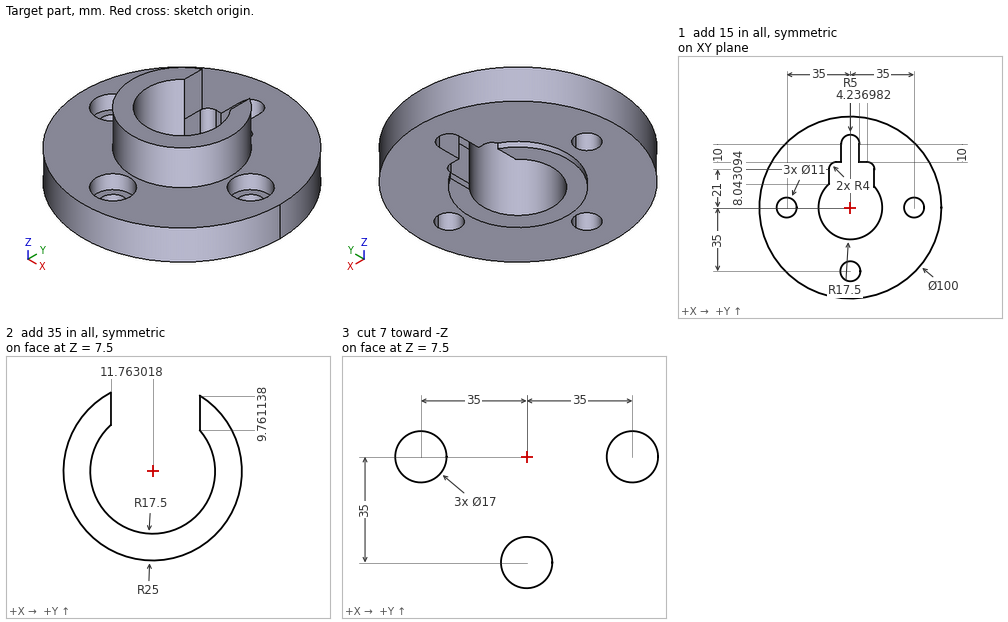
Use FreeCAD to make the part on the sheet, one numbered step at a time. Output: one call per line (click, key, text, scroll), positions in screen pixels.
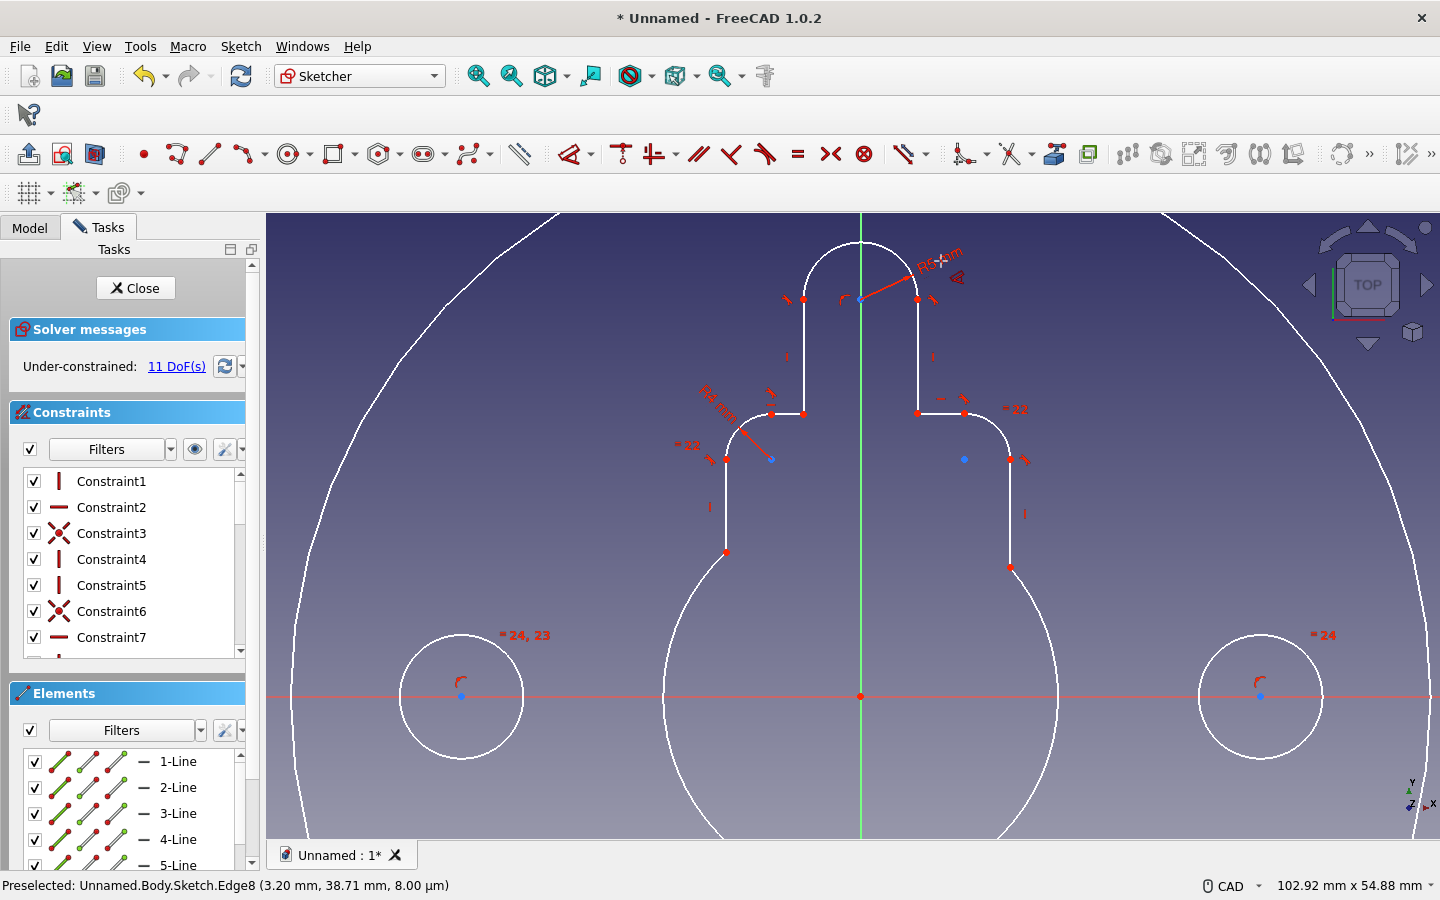
click(696, 805)
click(632, 715)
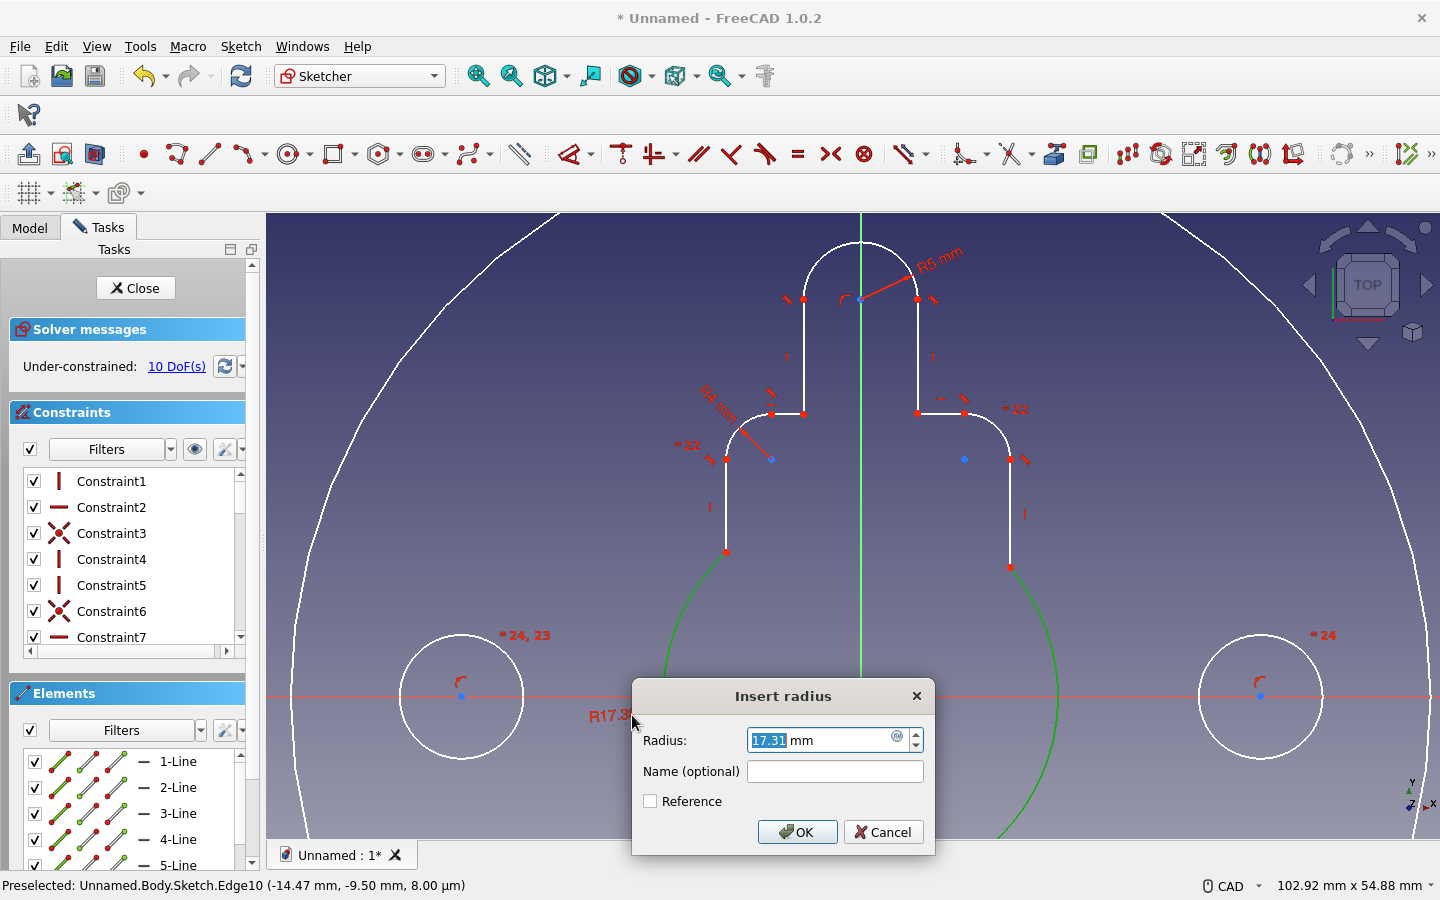
text(17.5)
key(Return)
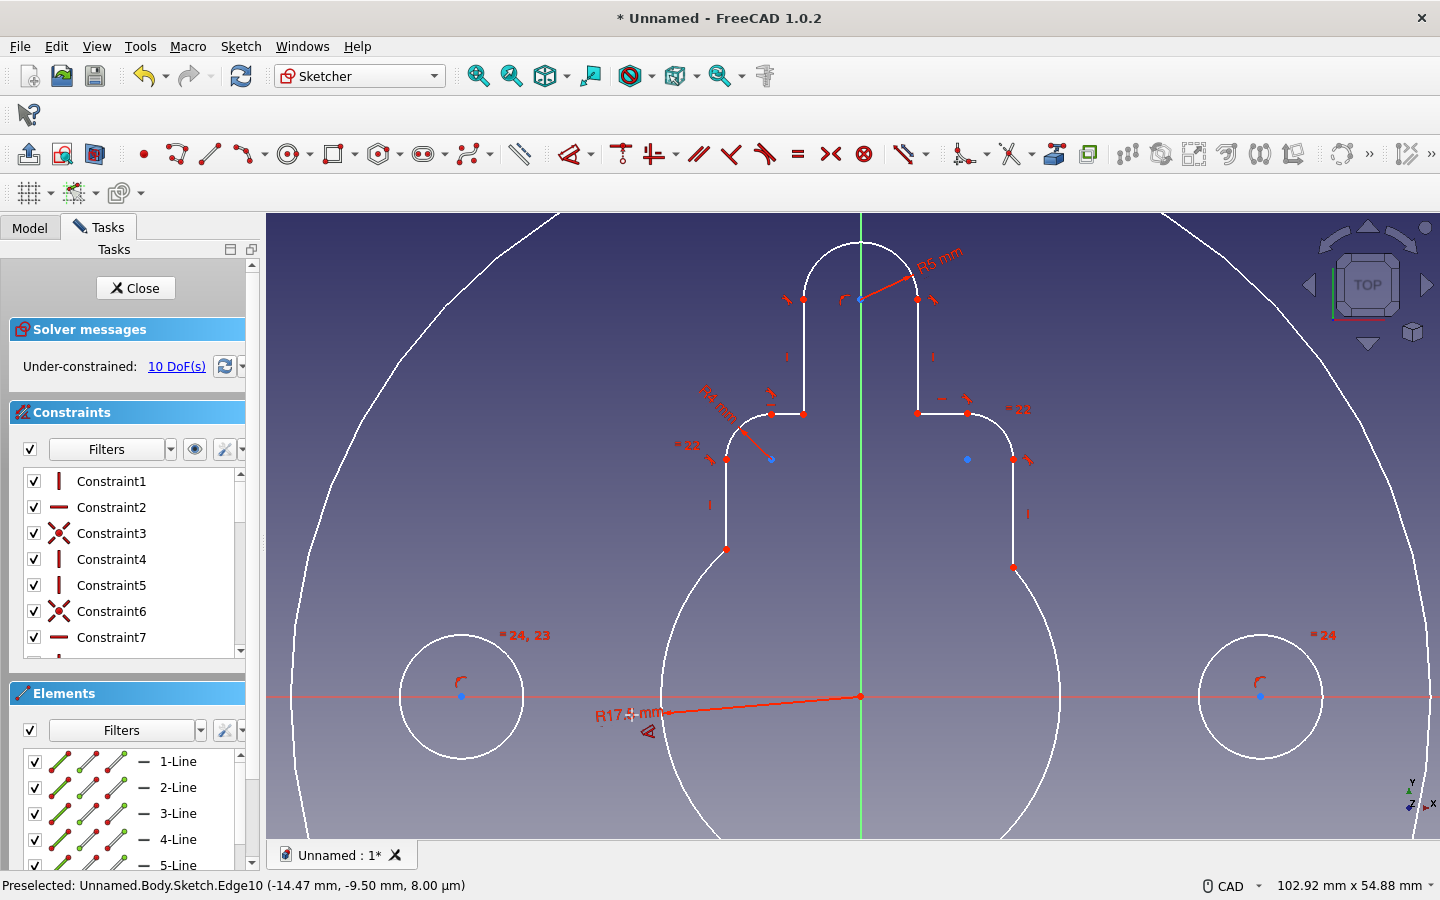
click(1262, 293)
click(434, 273)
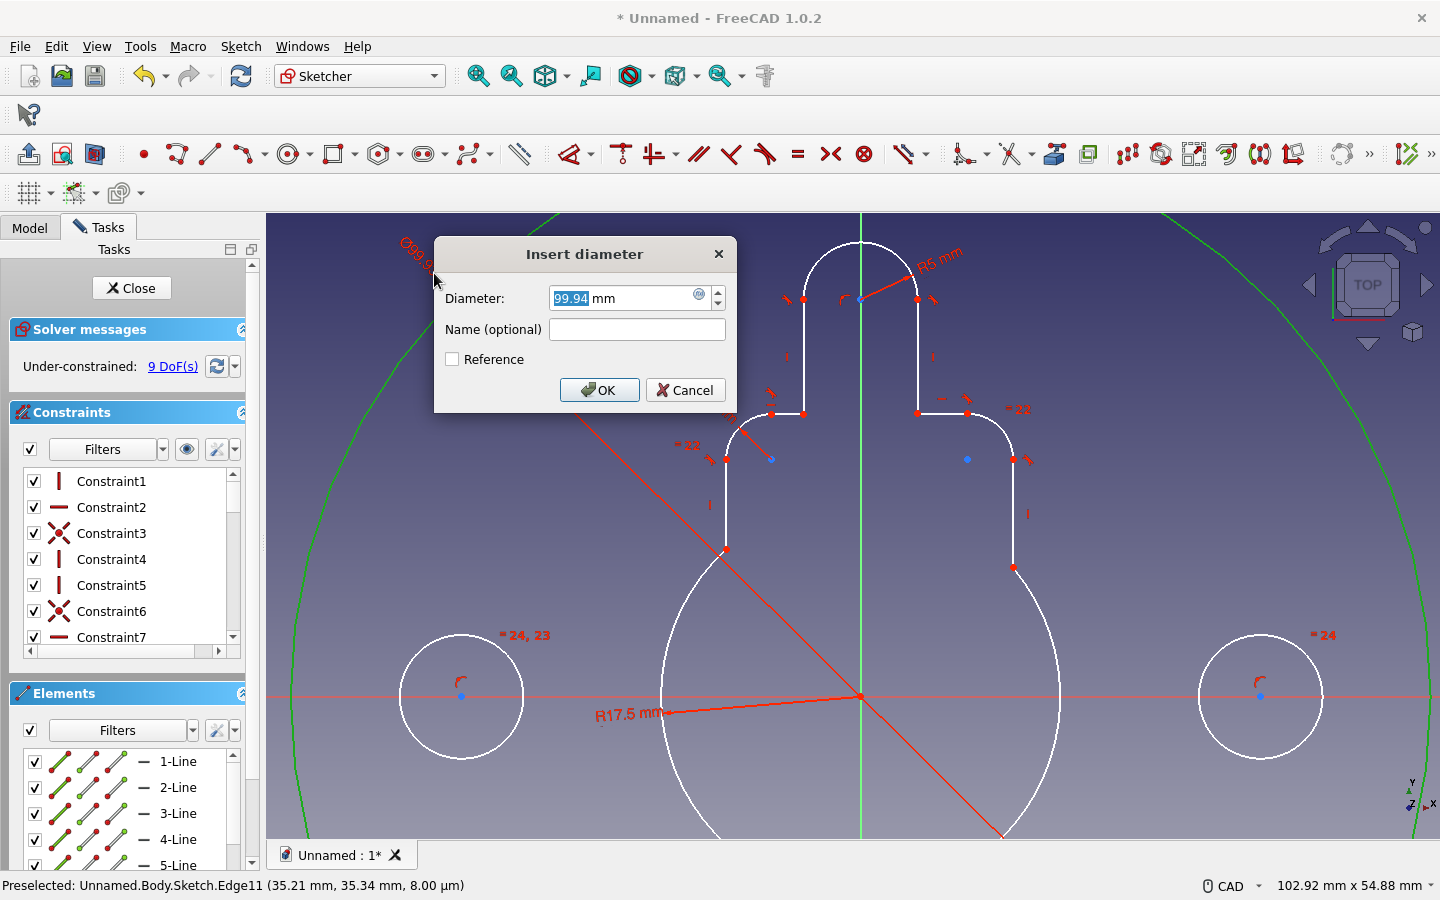
text(100)
key(Return)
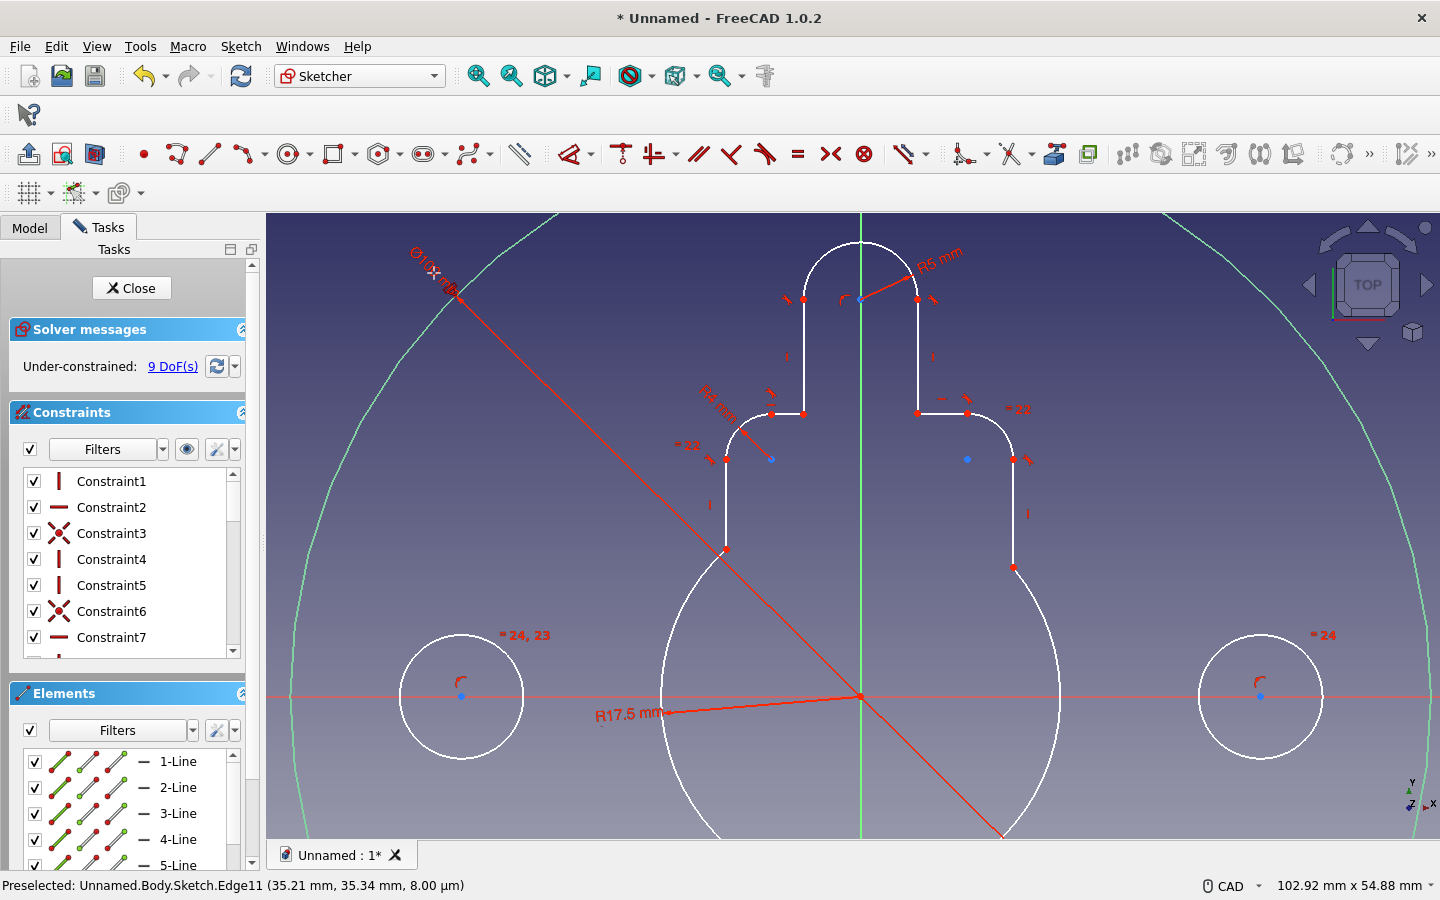
scroll(740, 427, down, 5)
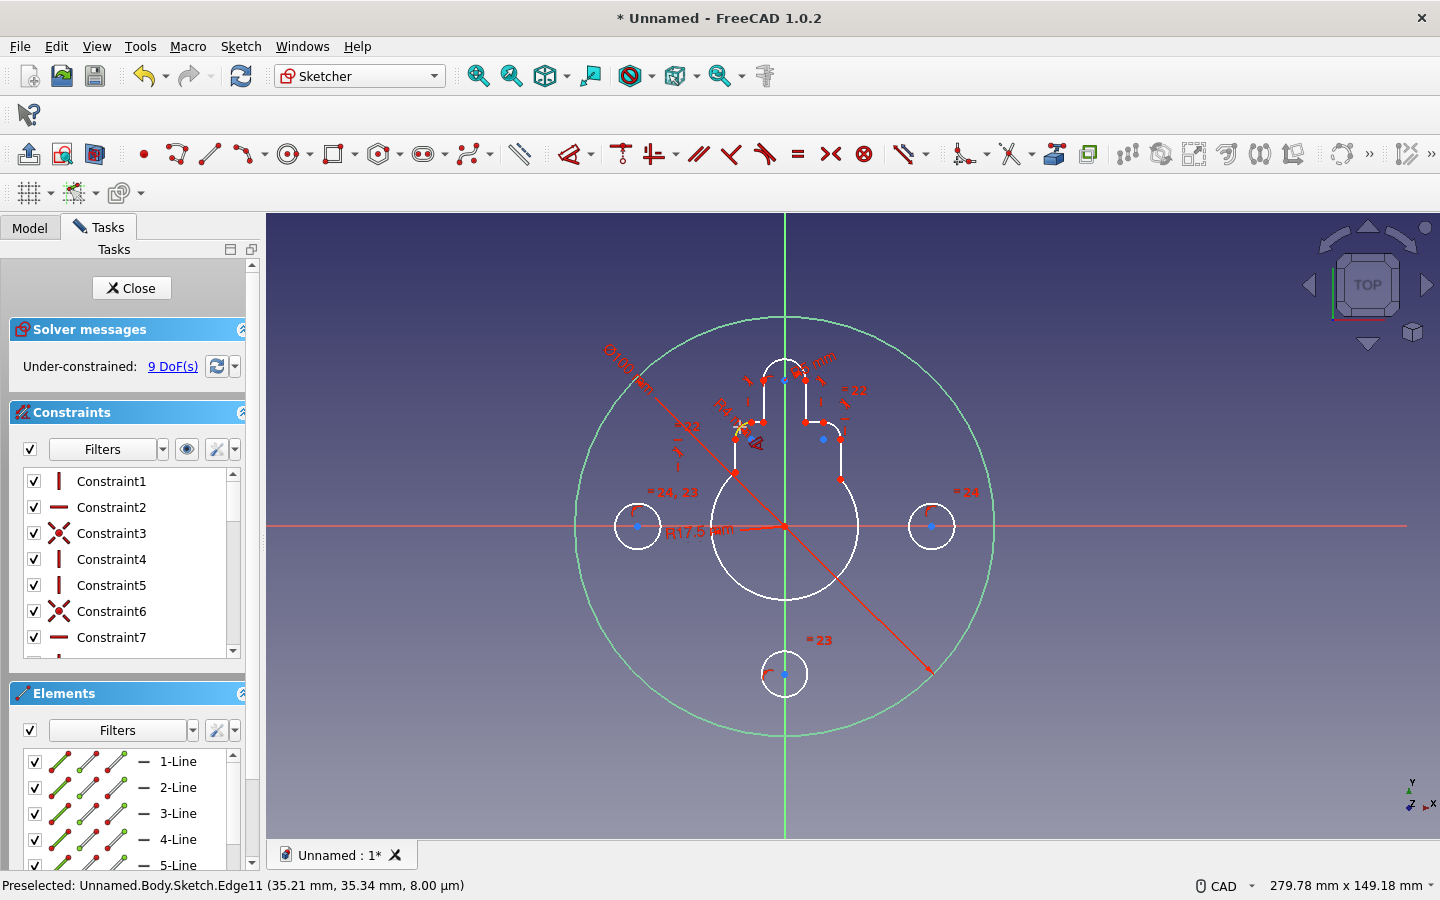
click(801, 658)
click(824, 636)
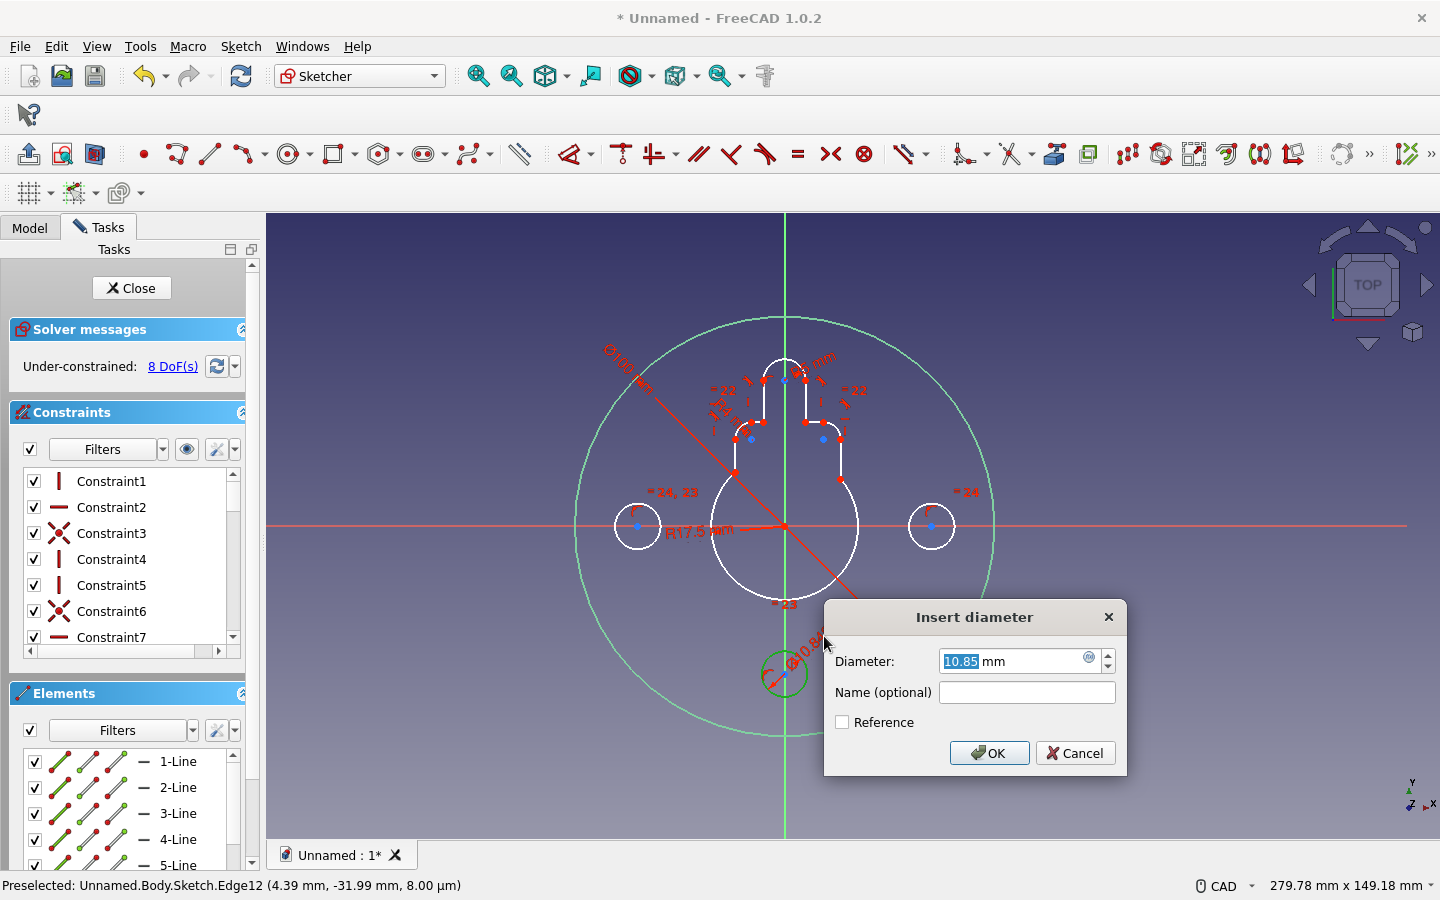
text(11)
key(Return)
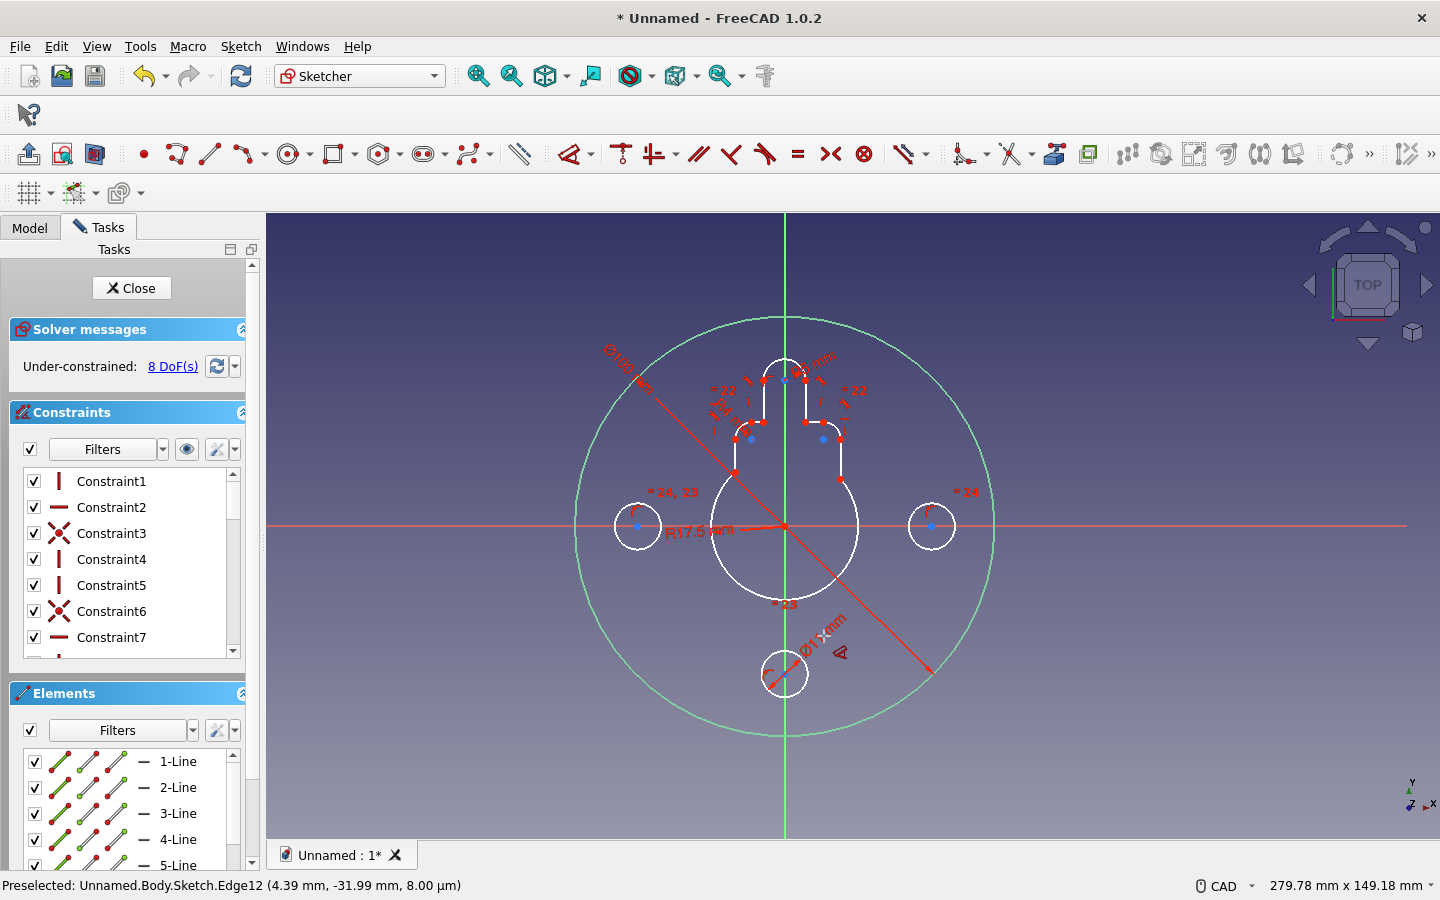
click(764, 410)
click(730, 392)